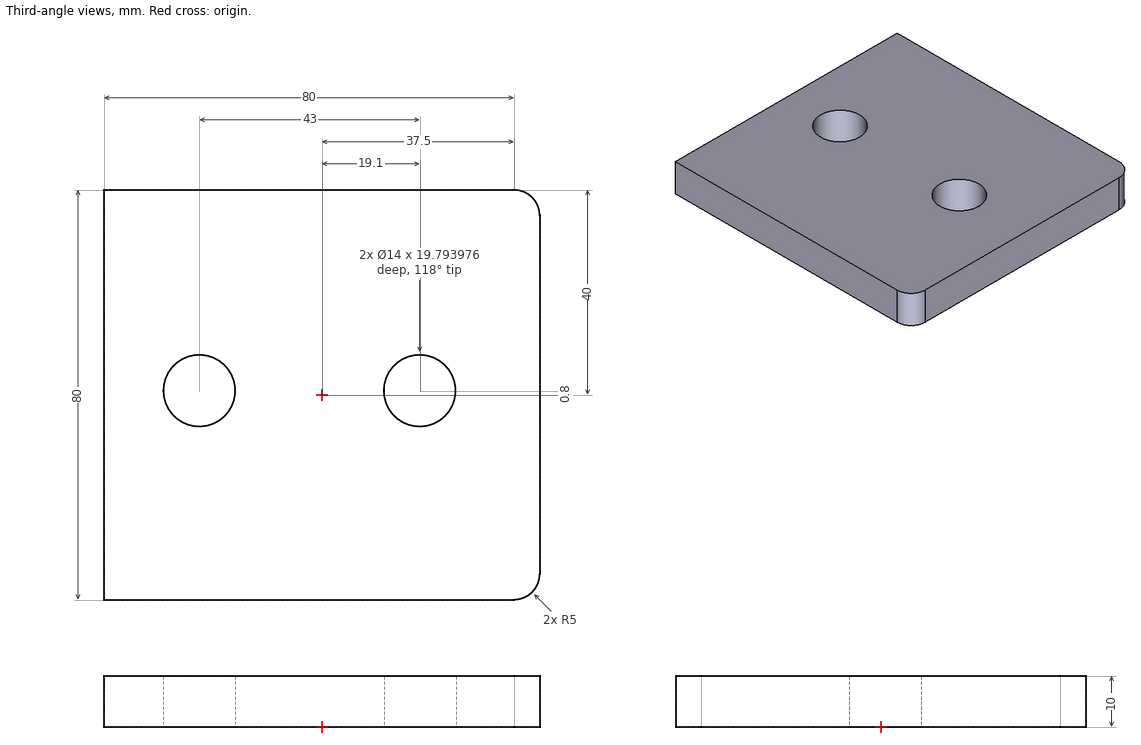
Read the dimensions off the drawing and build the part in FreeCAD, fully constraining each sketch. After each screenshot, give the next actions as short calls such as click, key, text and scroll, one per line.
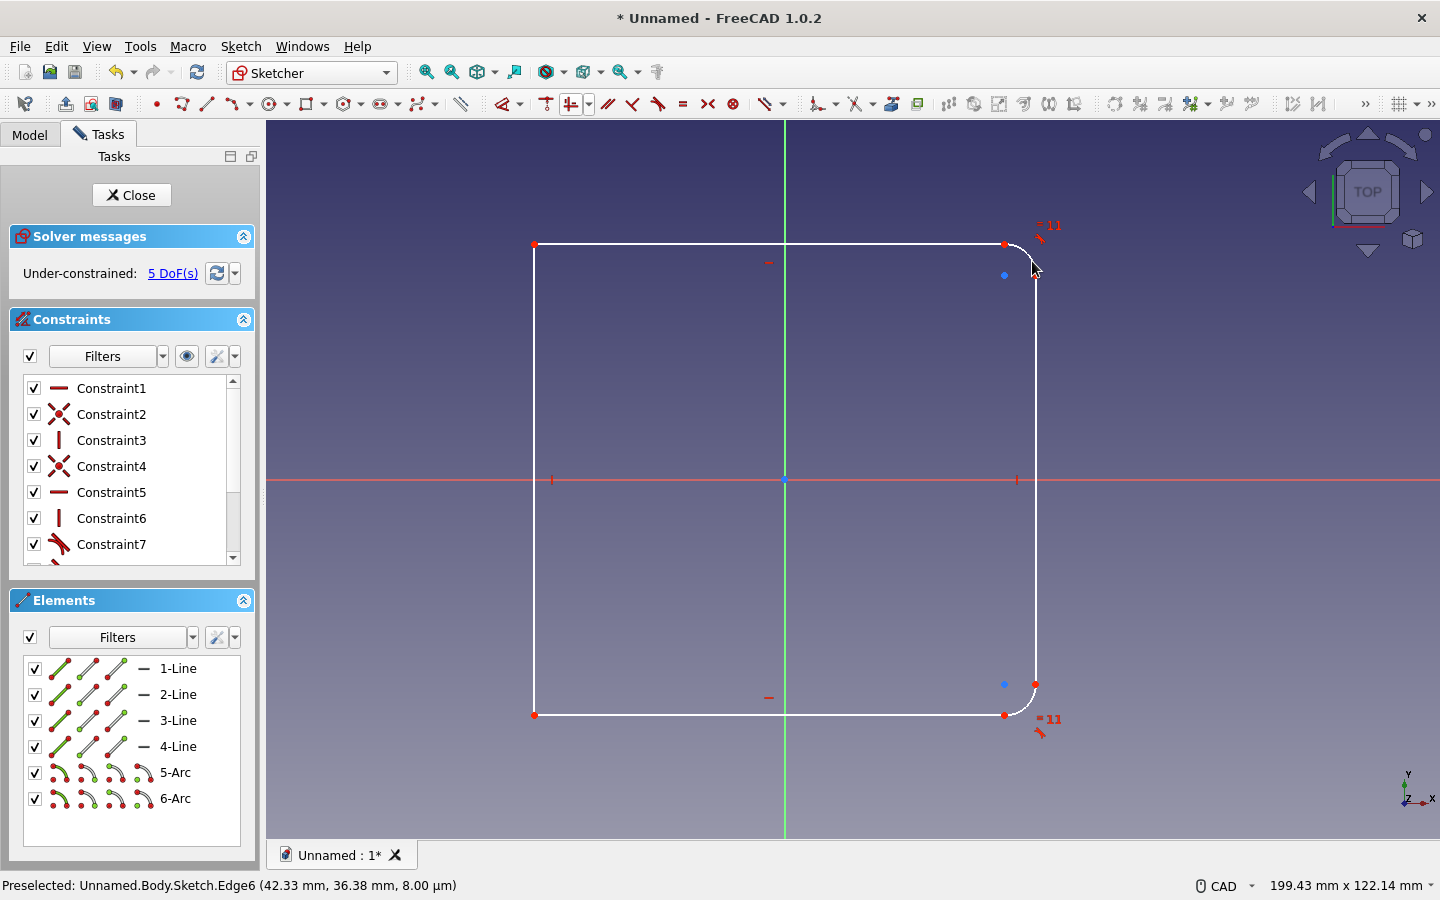
scroll(1019, 712, up, 2)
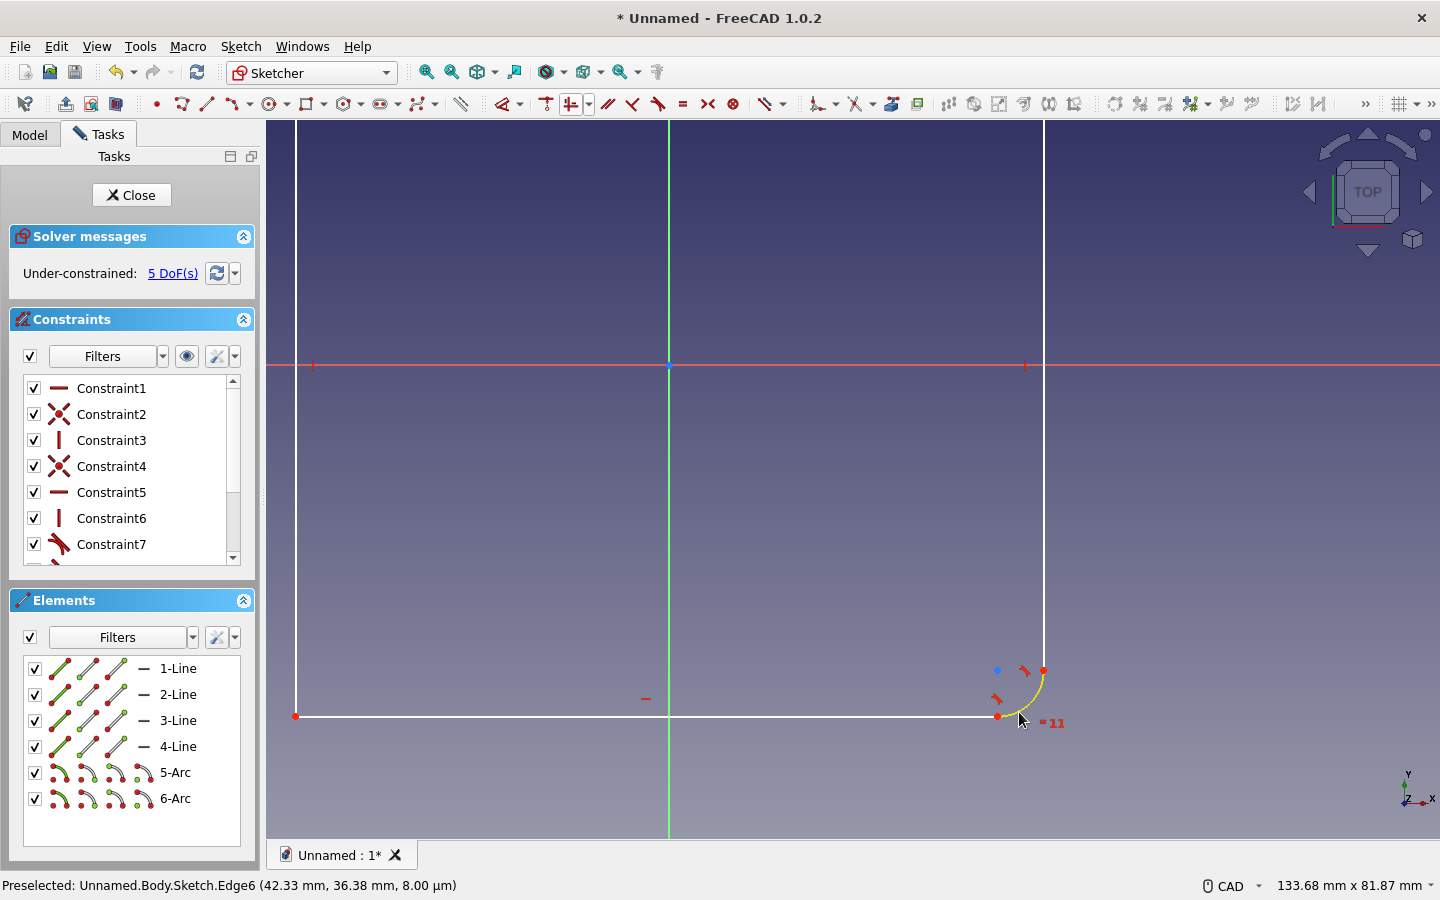
click(1019, 712)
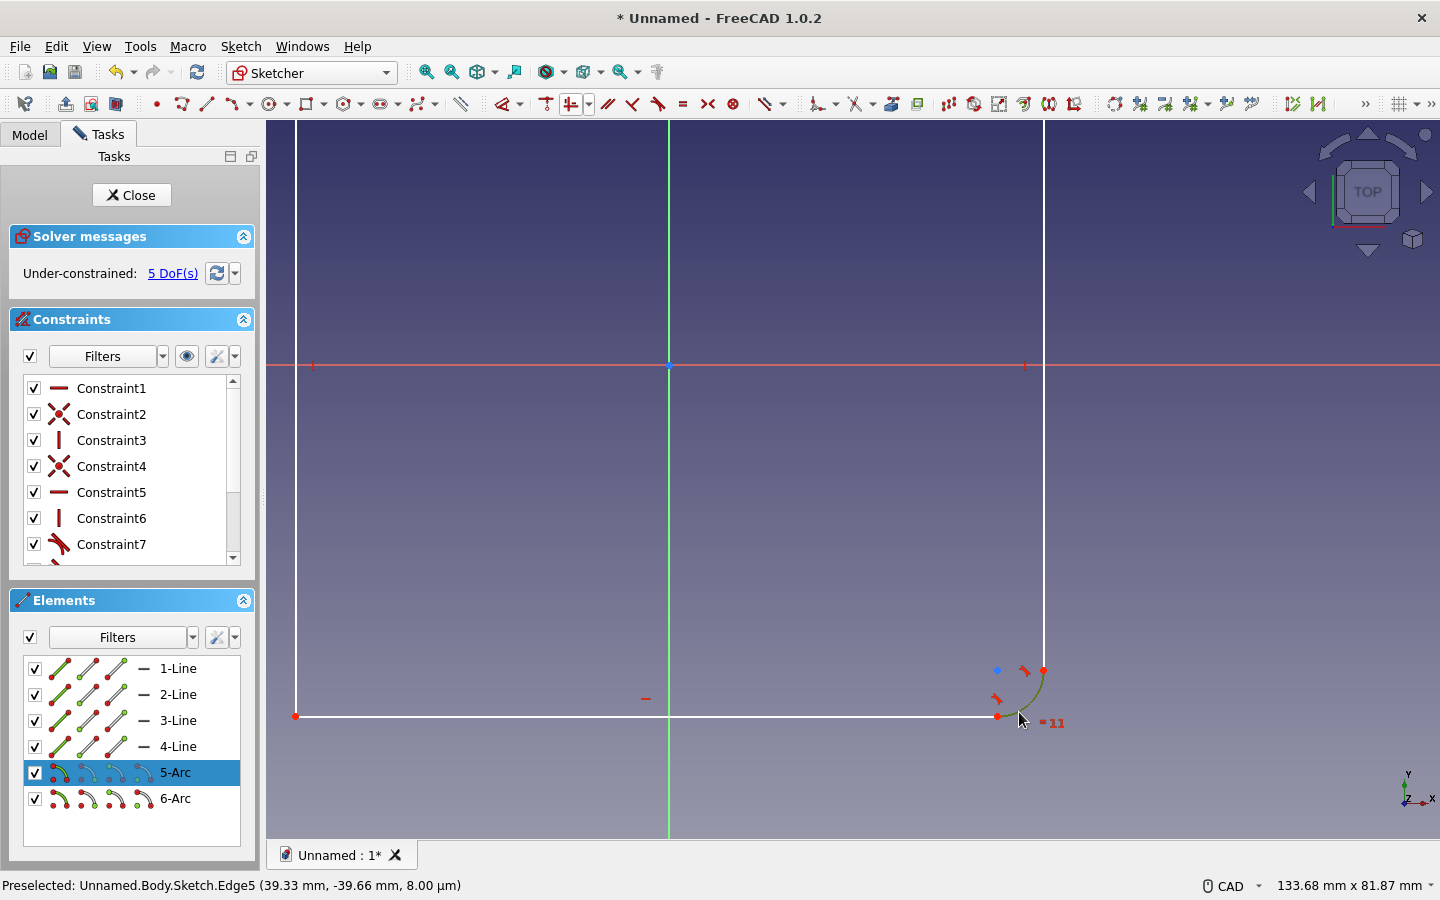
click(520, 104)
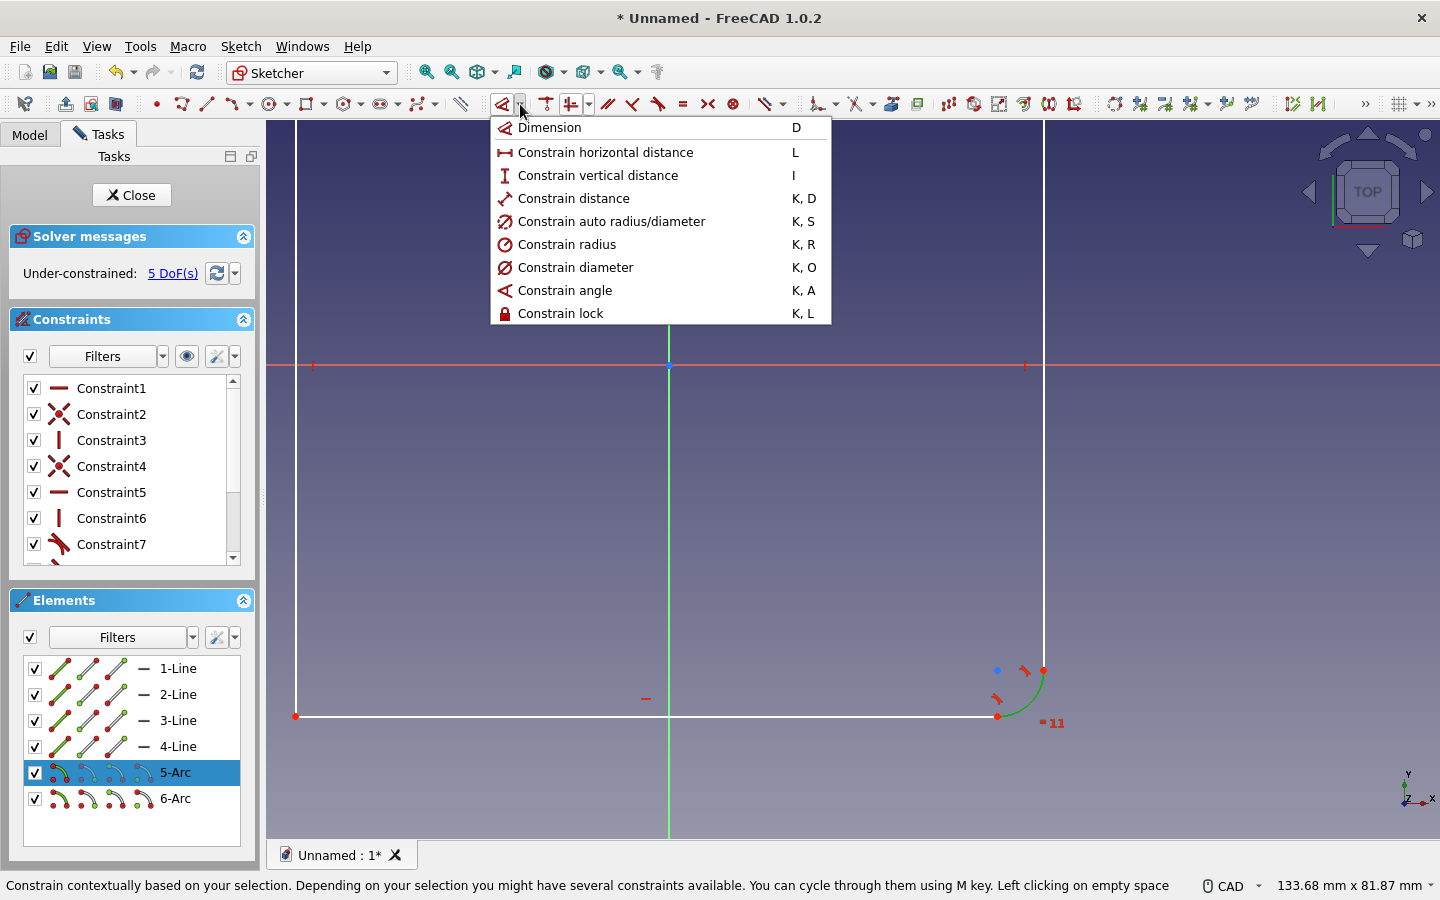
click(661, 244)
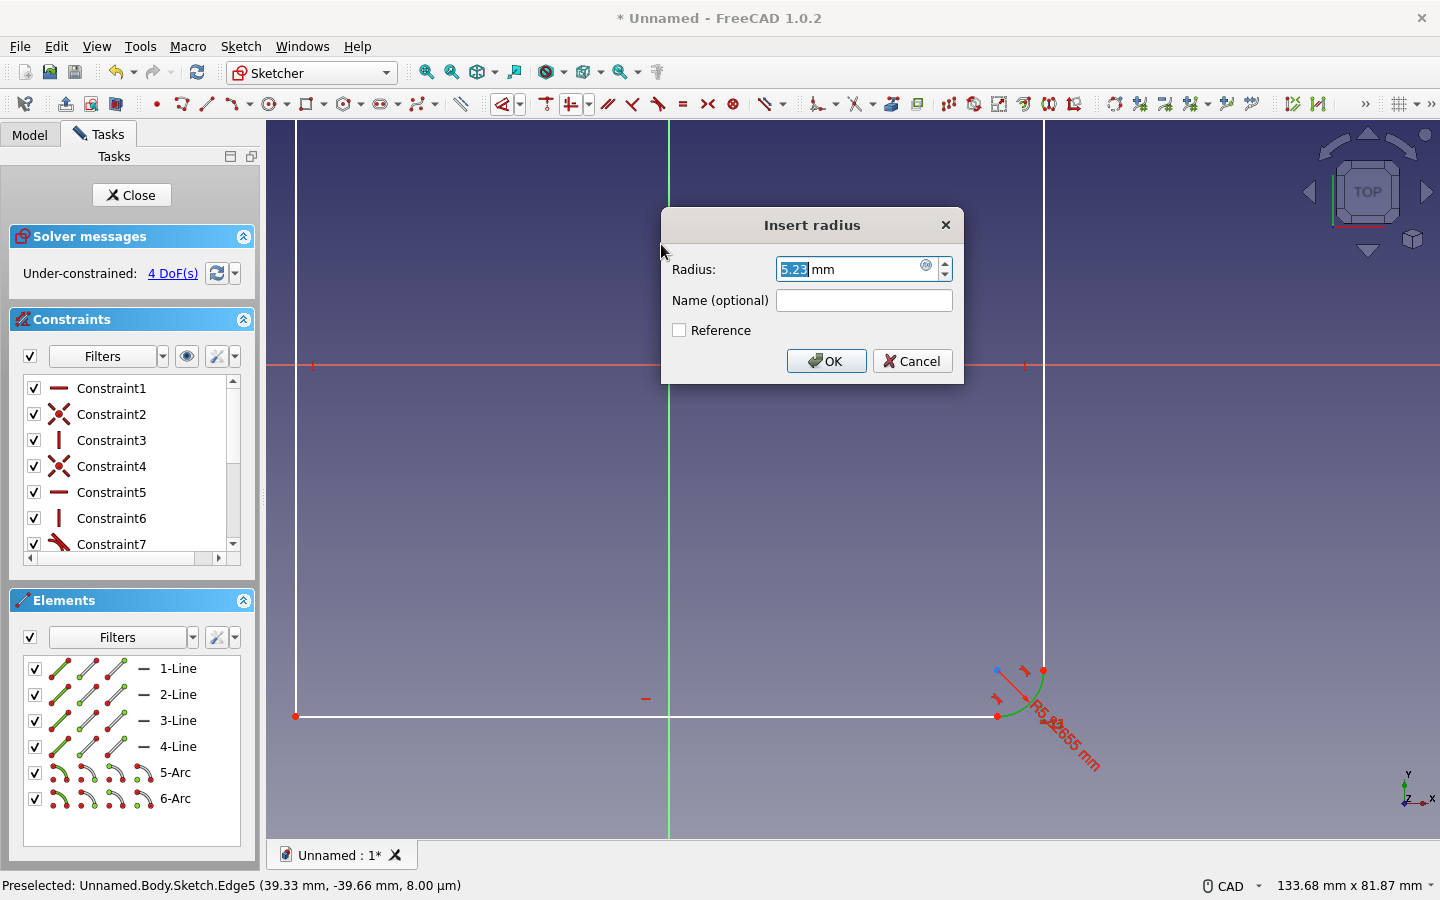
text(5)
key(Return)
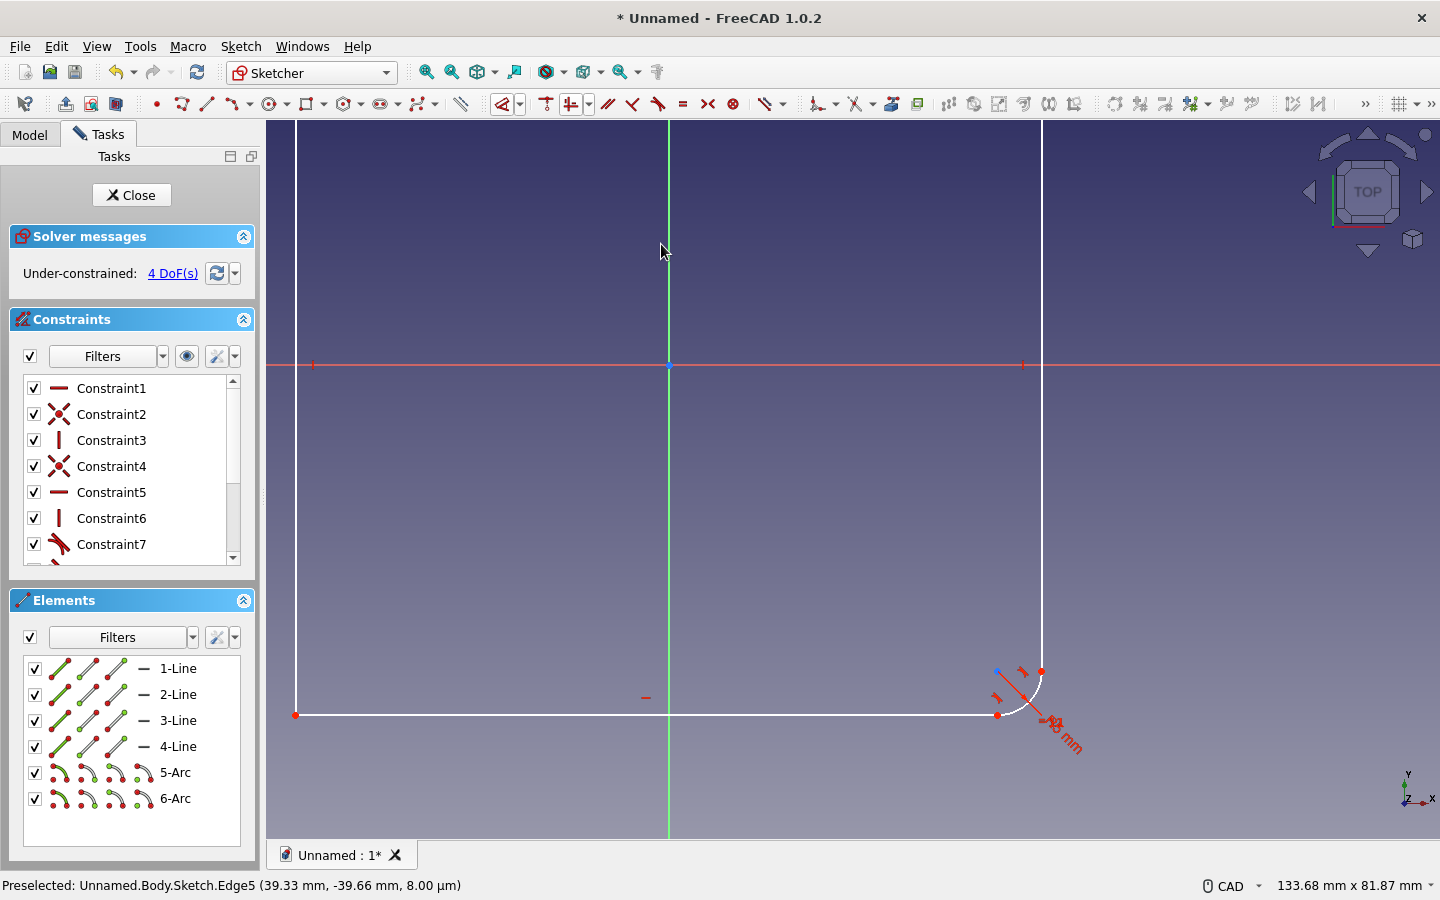
scroll(1019, 712, down, 2)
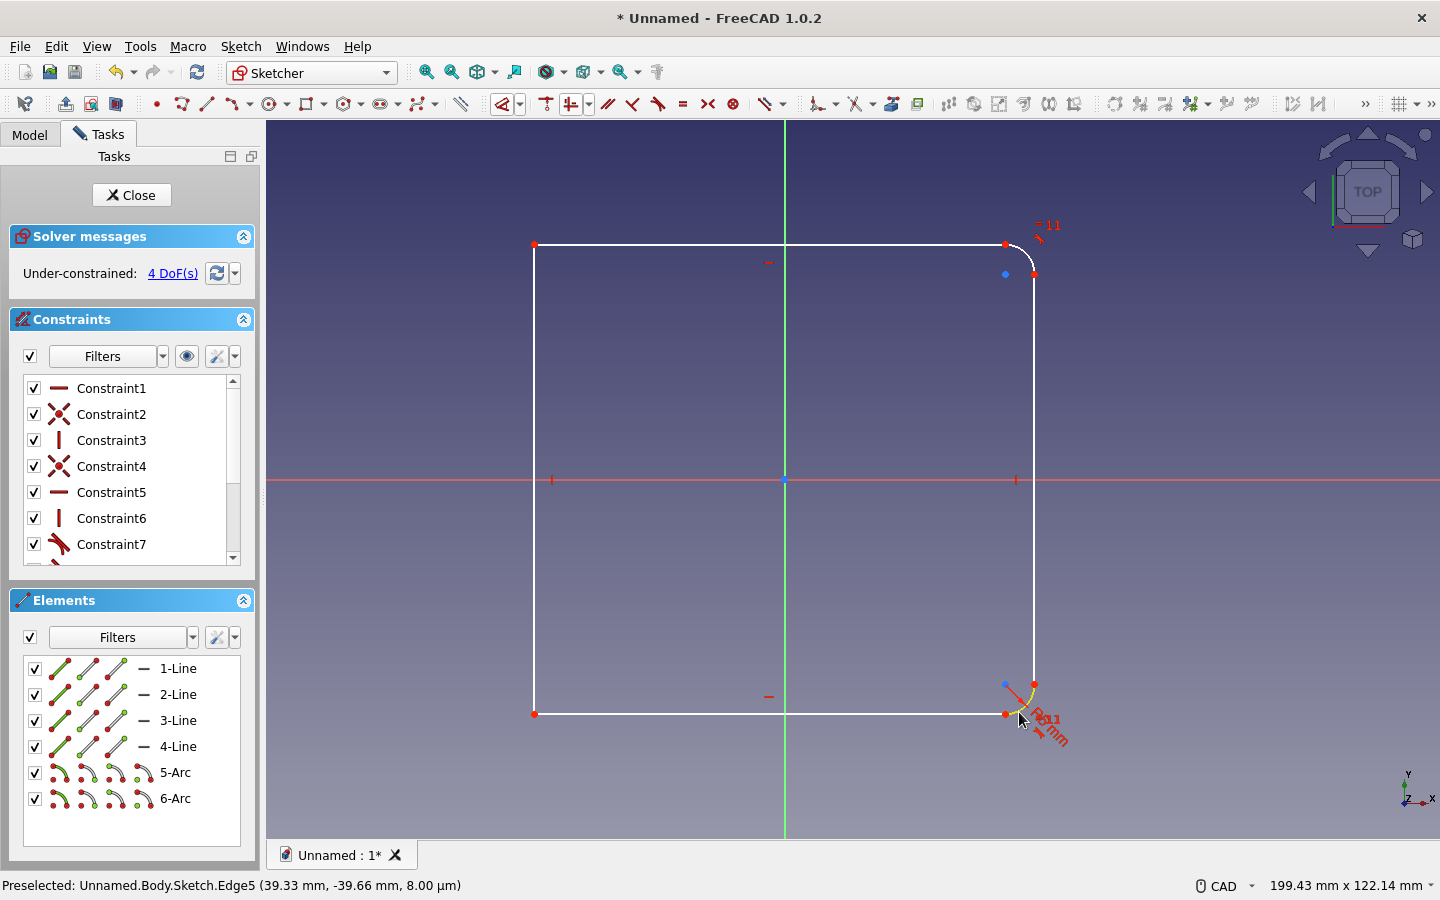
click(864, 245)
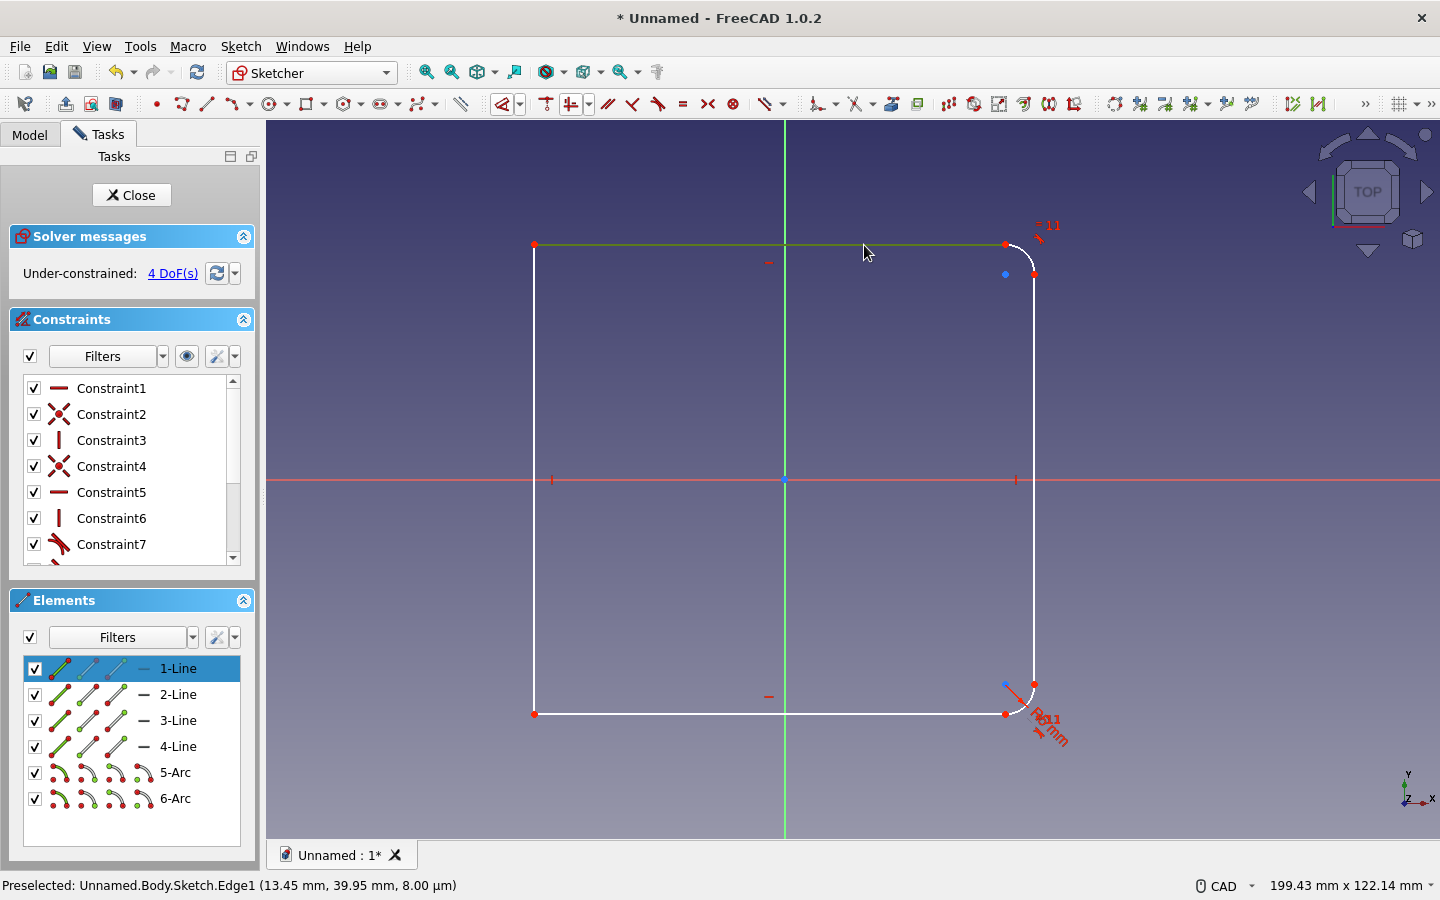
key(l)